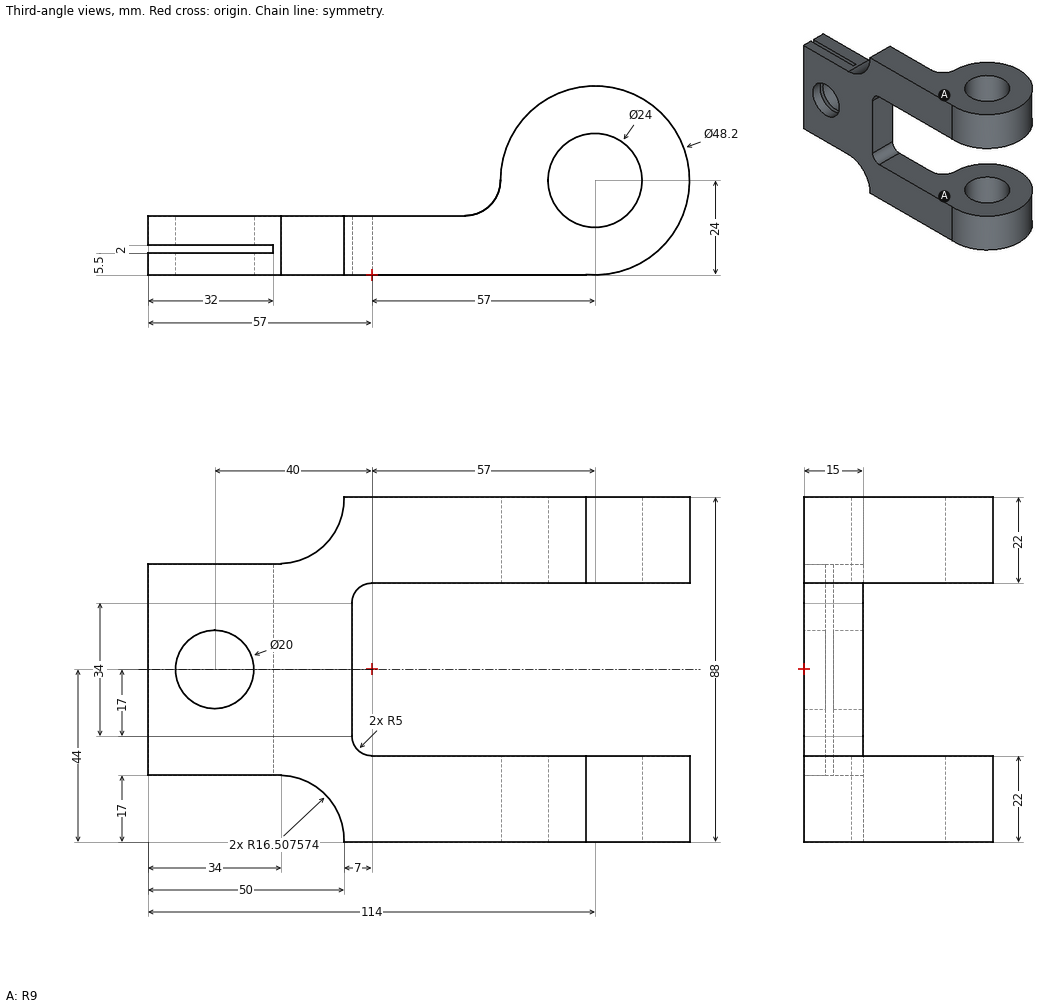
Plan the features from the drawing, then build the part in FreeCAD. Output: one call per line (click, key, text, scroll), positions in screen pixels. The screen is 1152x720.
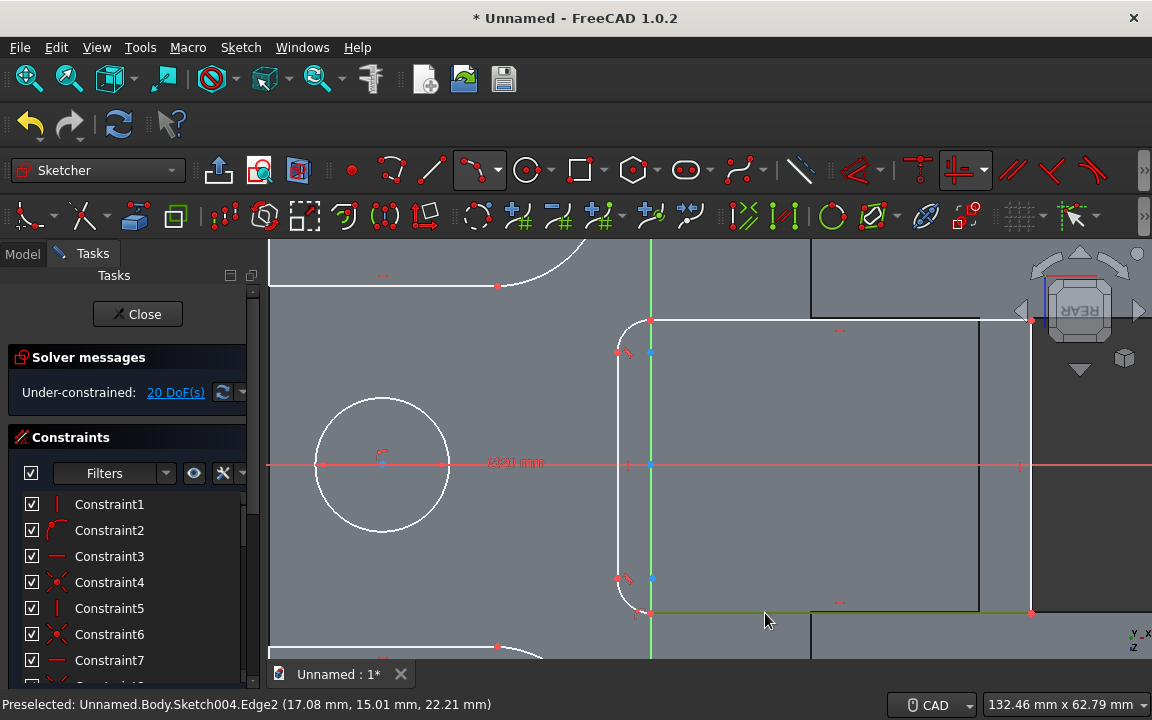
click(621, 594)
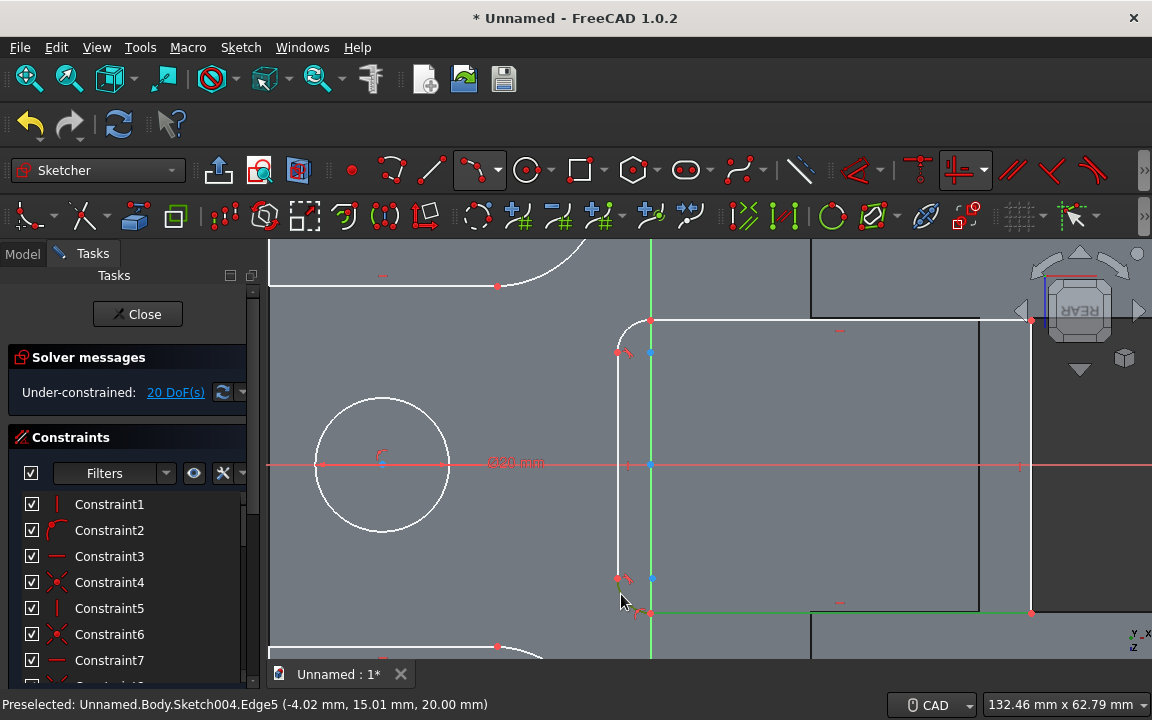
click(1094, 170)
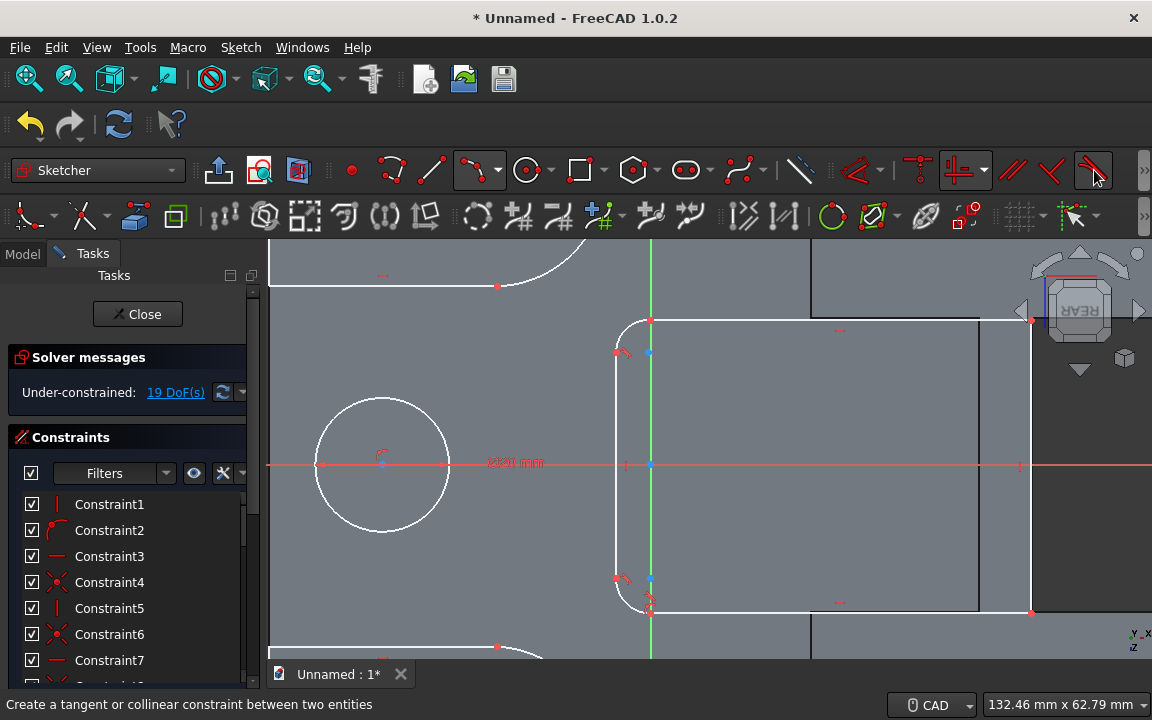
click(917, 320)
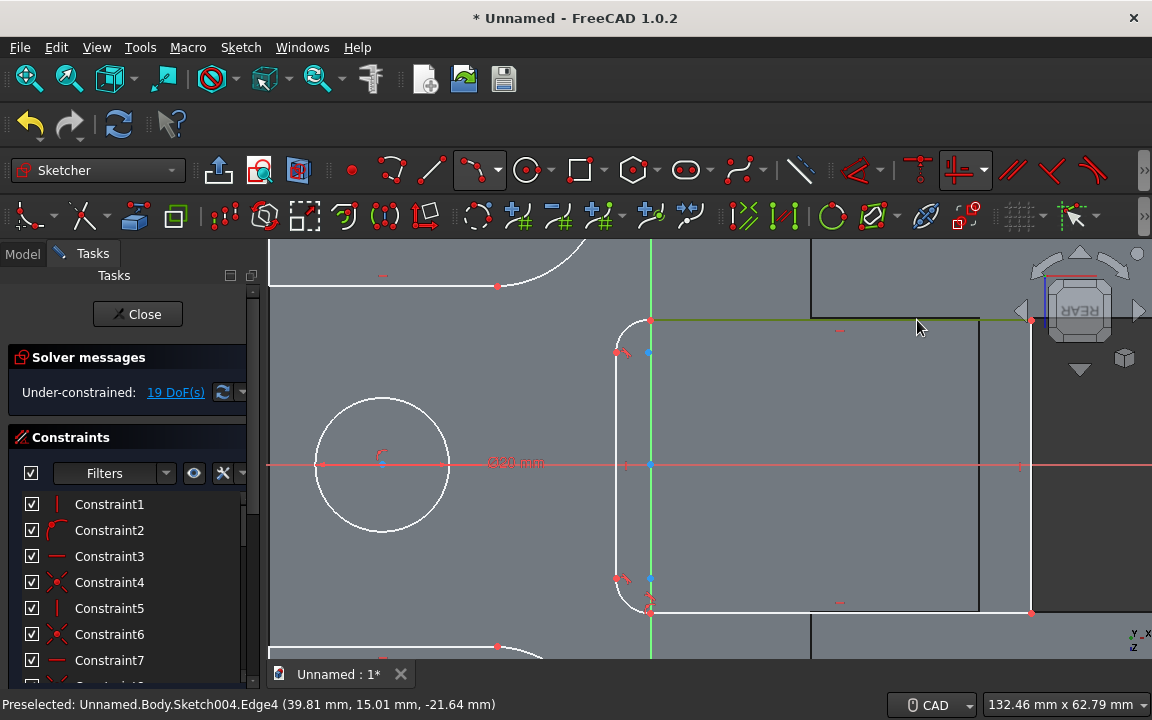
click(635, 323)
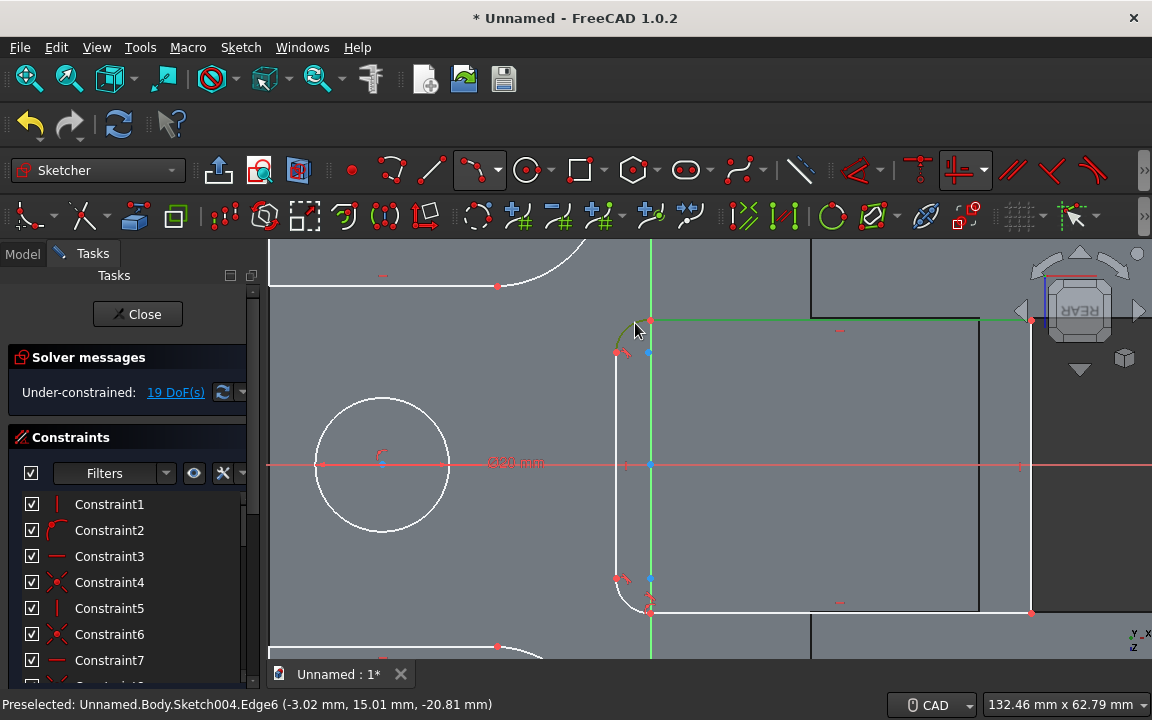
key(t)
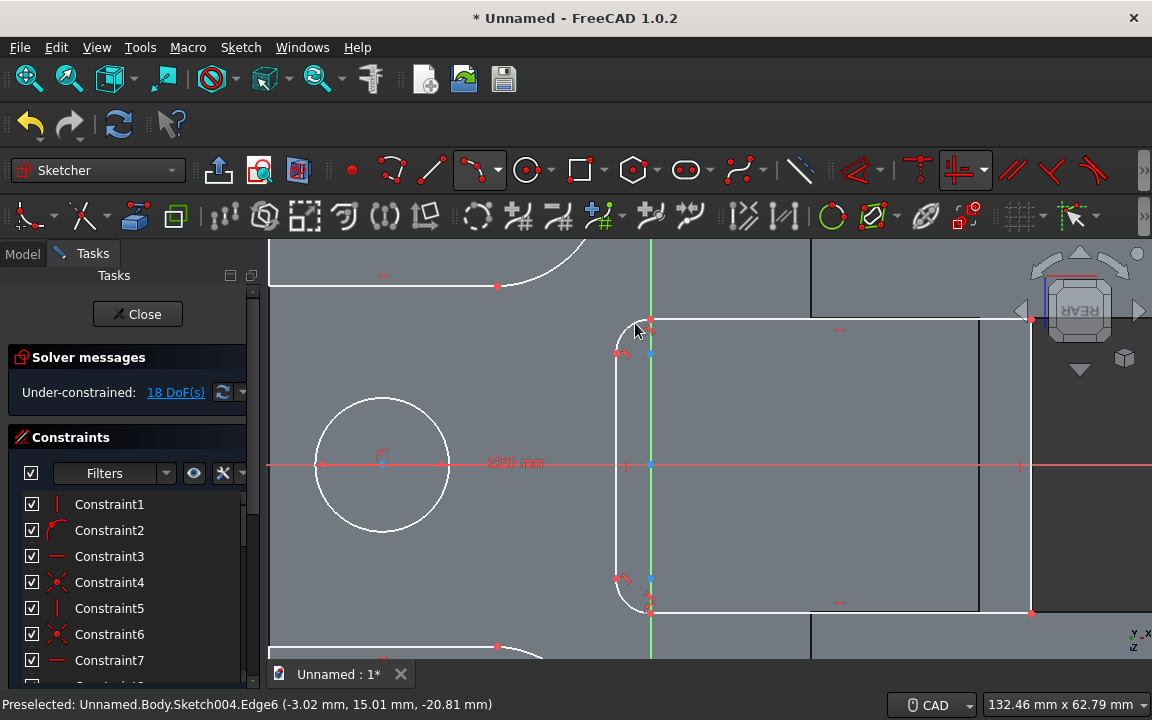
click(620, 594)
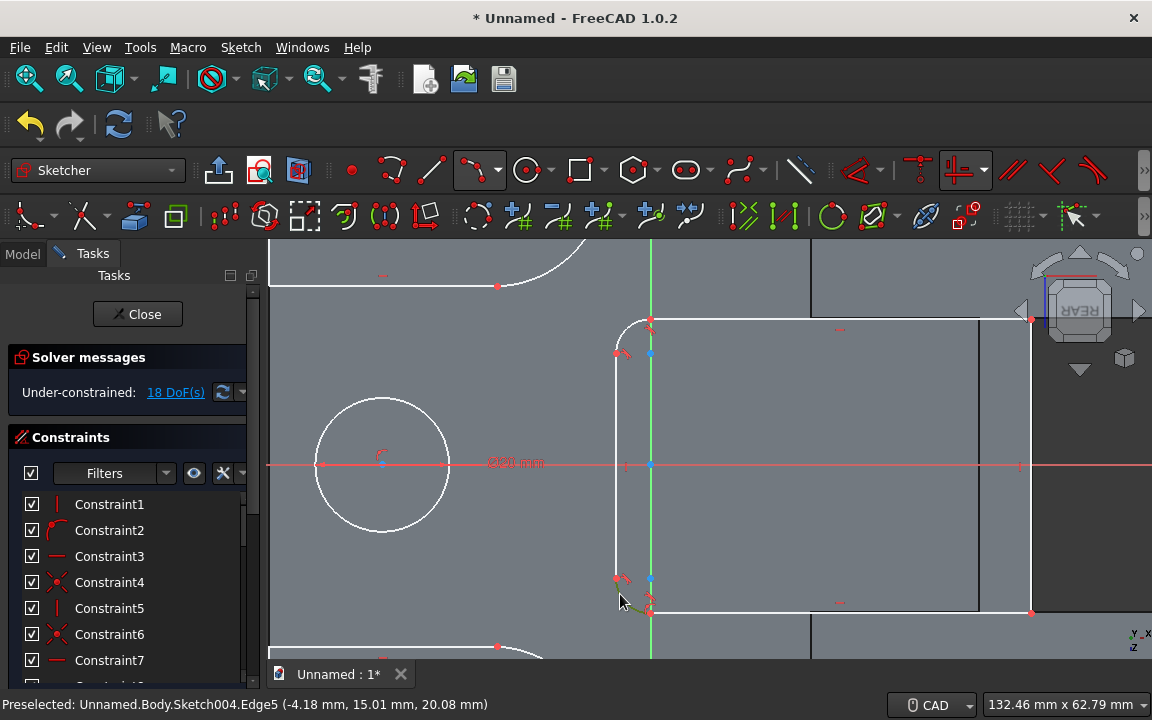
click(635, 323)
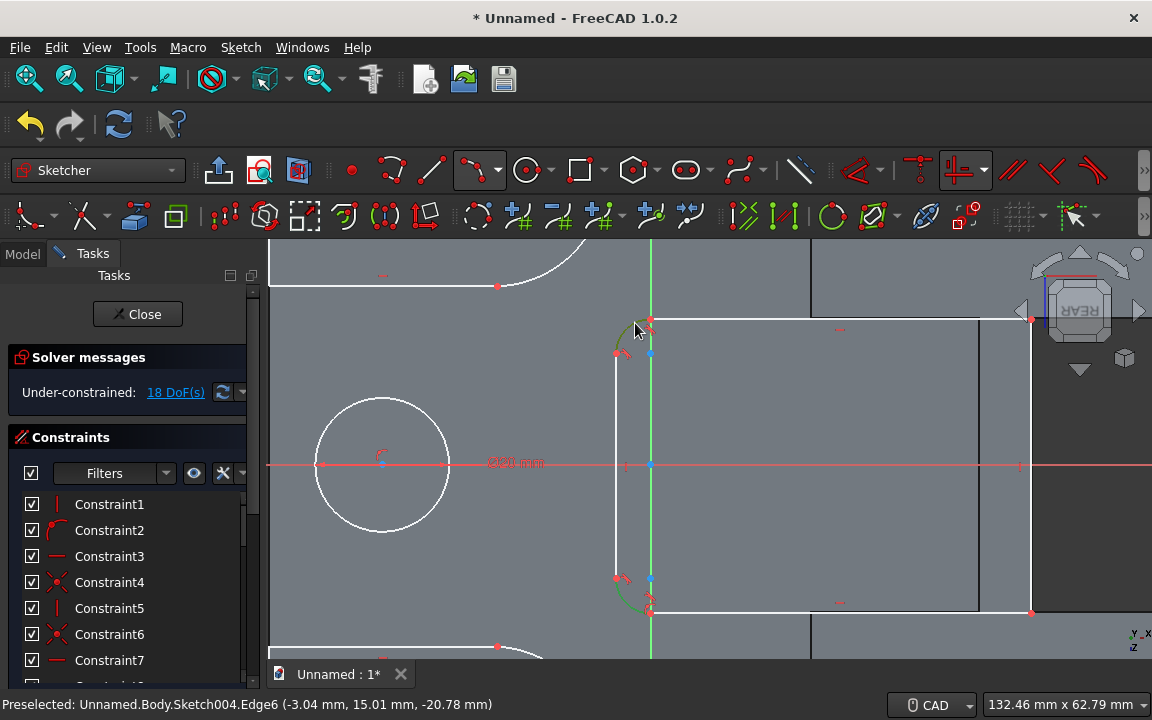
key(e)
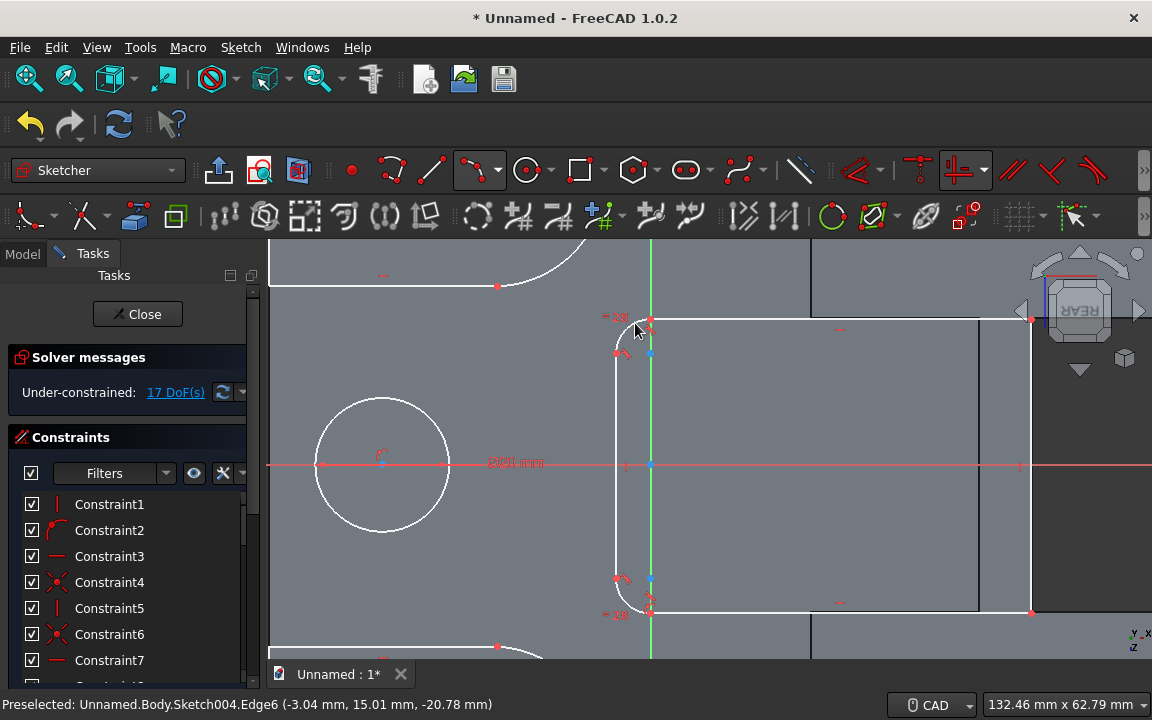
click(548, 273)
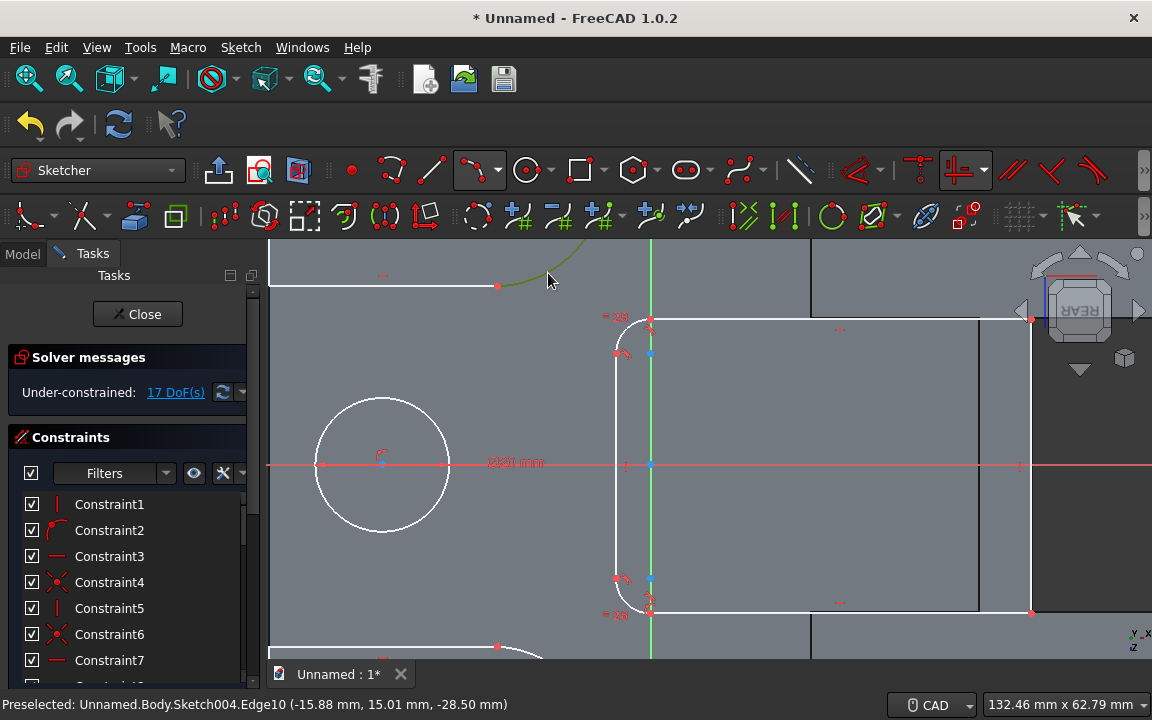
scroll(632, 436, down, 4)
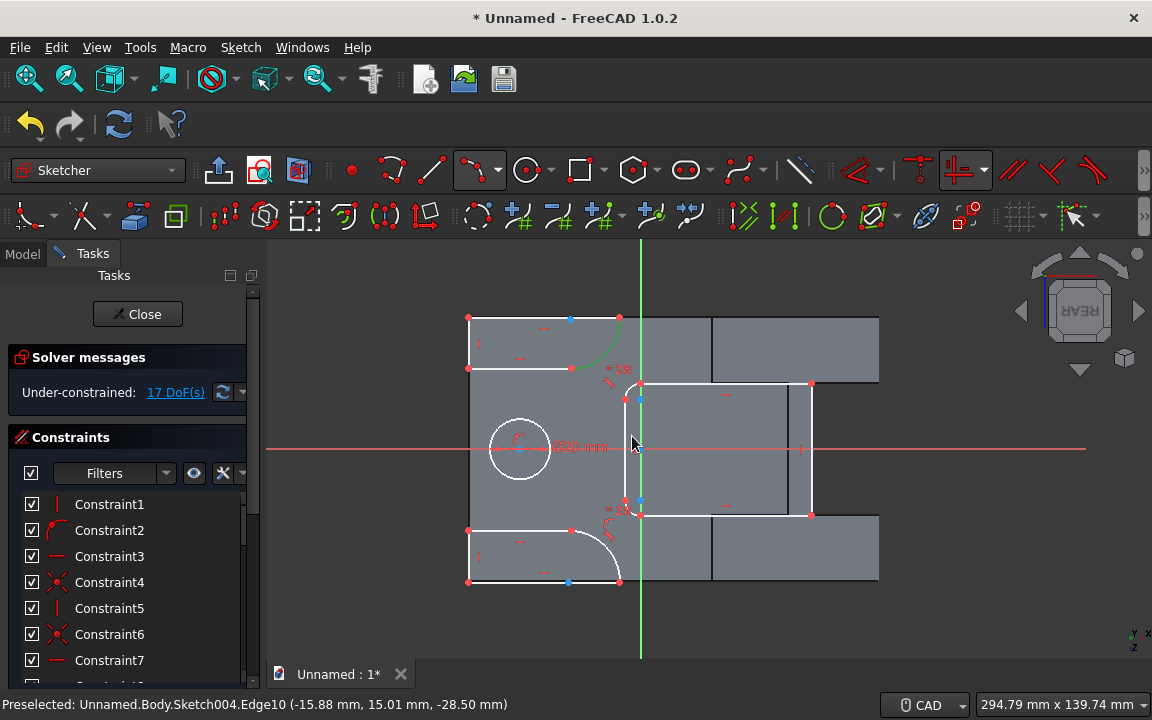
click(615, 560)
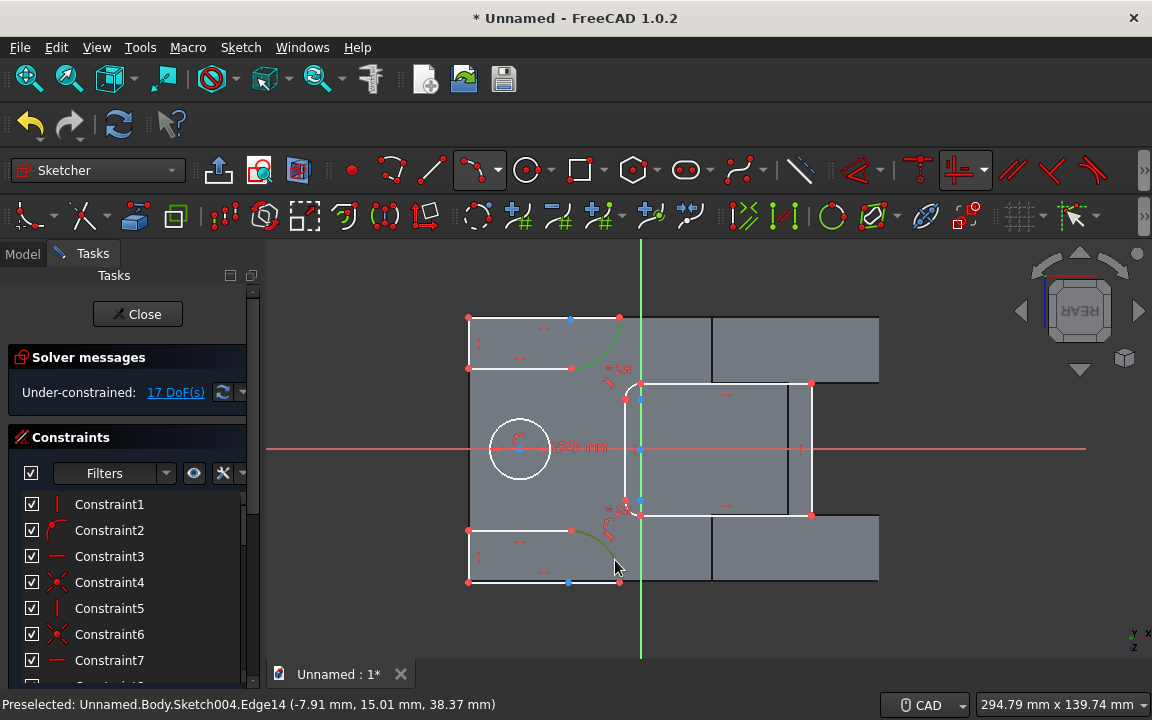
key(e)